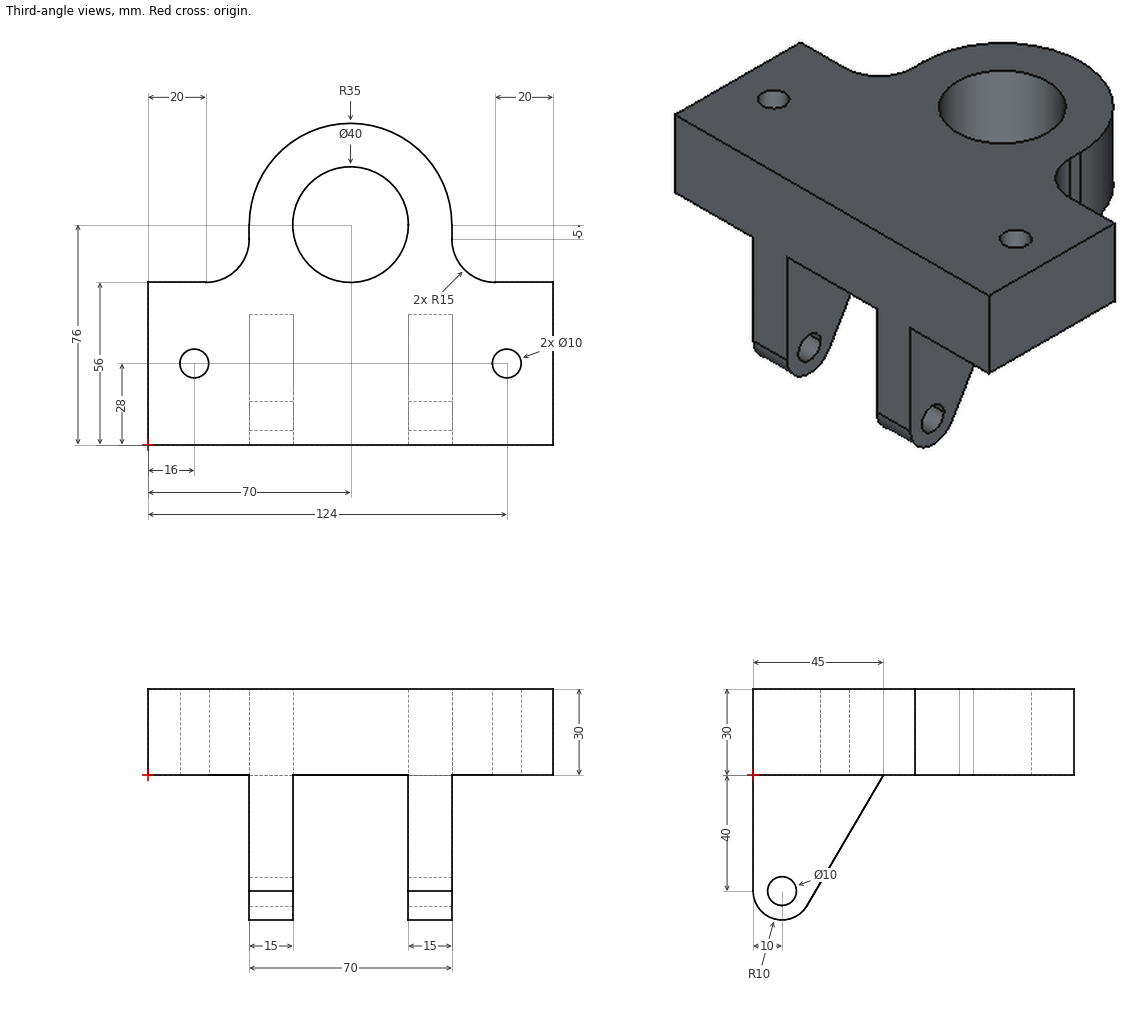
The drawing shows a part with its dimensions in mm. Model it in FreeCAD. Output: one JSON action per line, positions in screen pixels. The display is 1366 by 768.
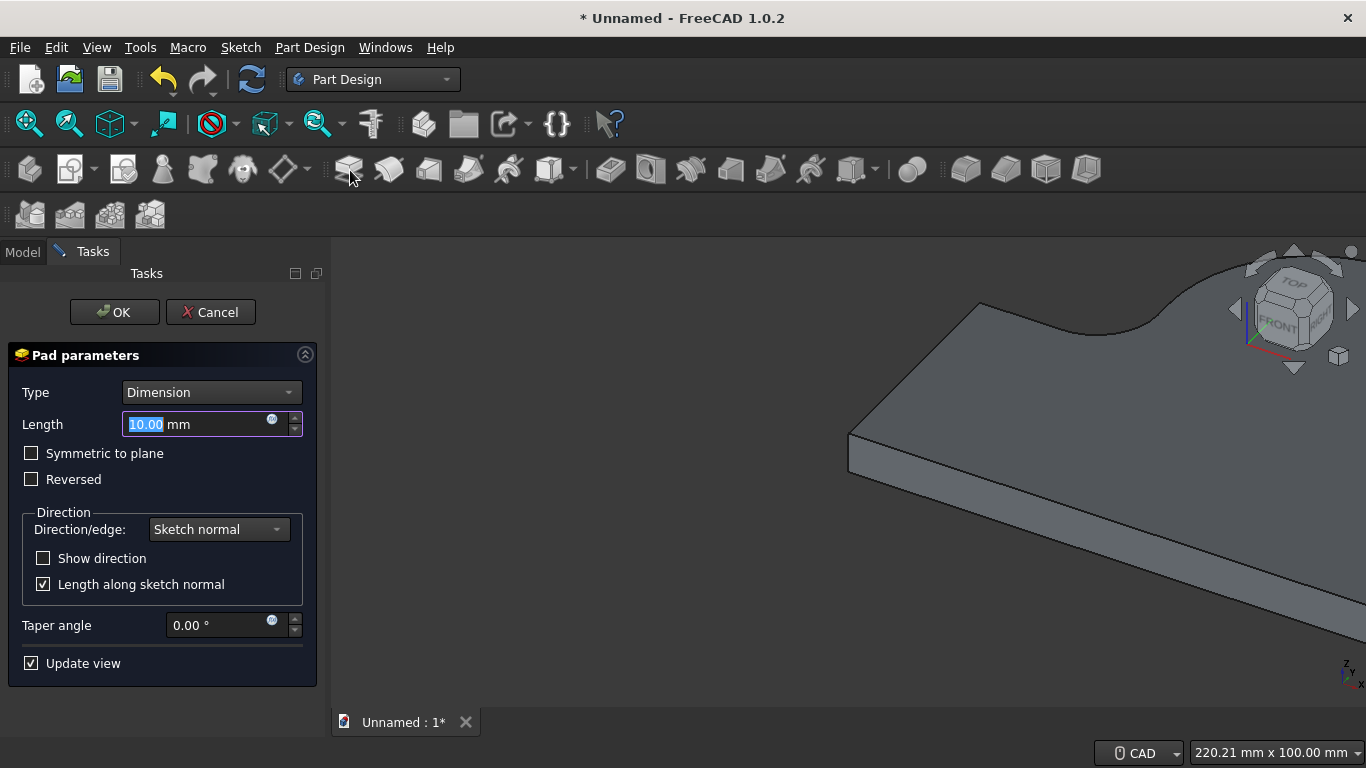
{"action": "type", "text": "30"}
{"action": "key", "text": "Tab"}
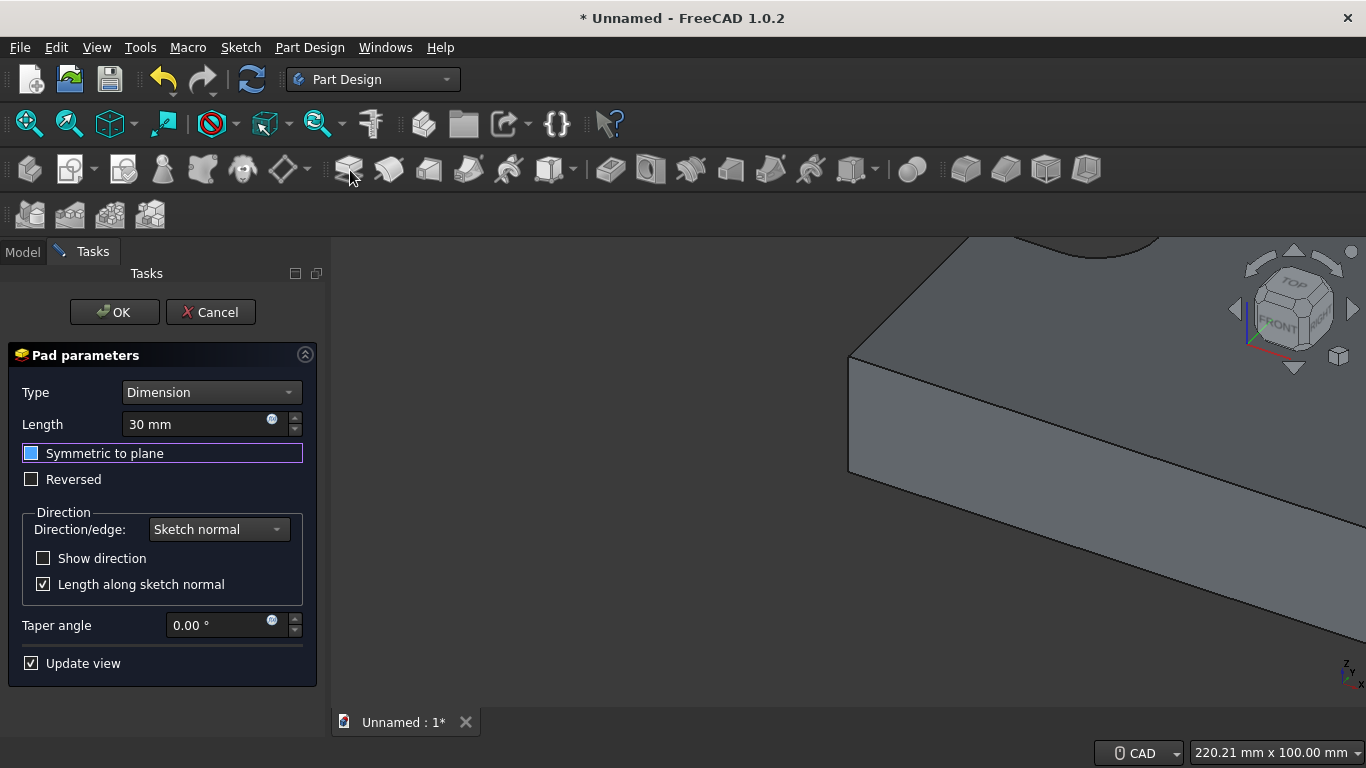
{"action": "left_click", "coordinate": [115, 312]}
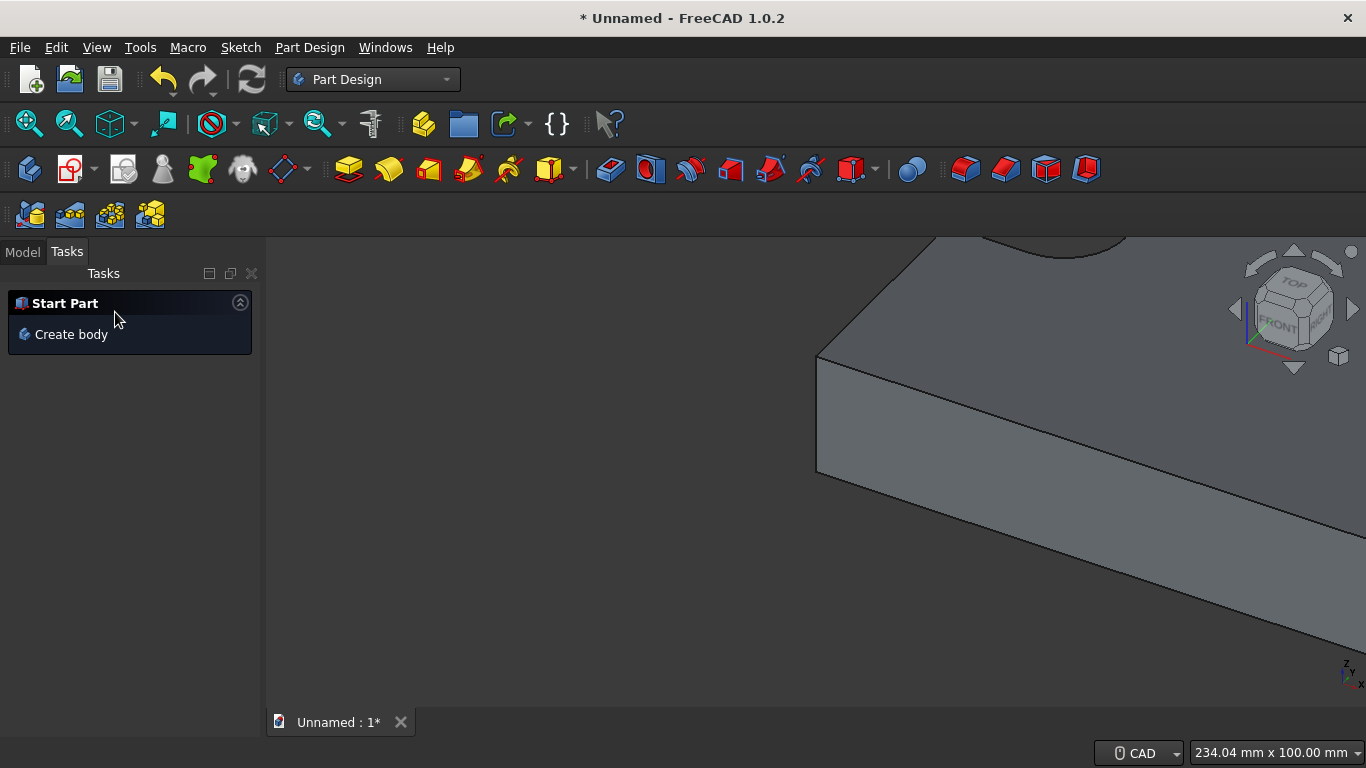
{"action": "left_click", "coordinate": [30, 124]}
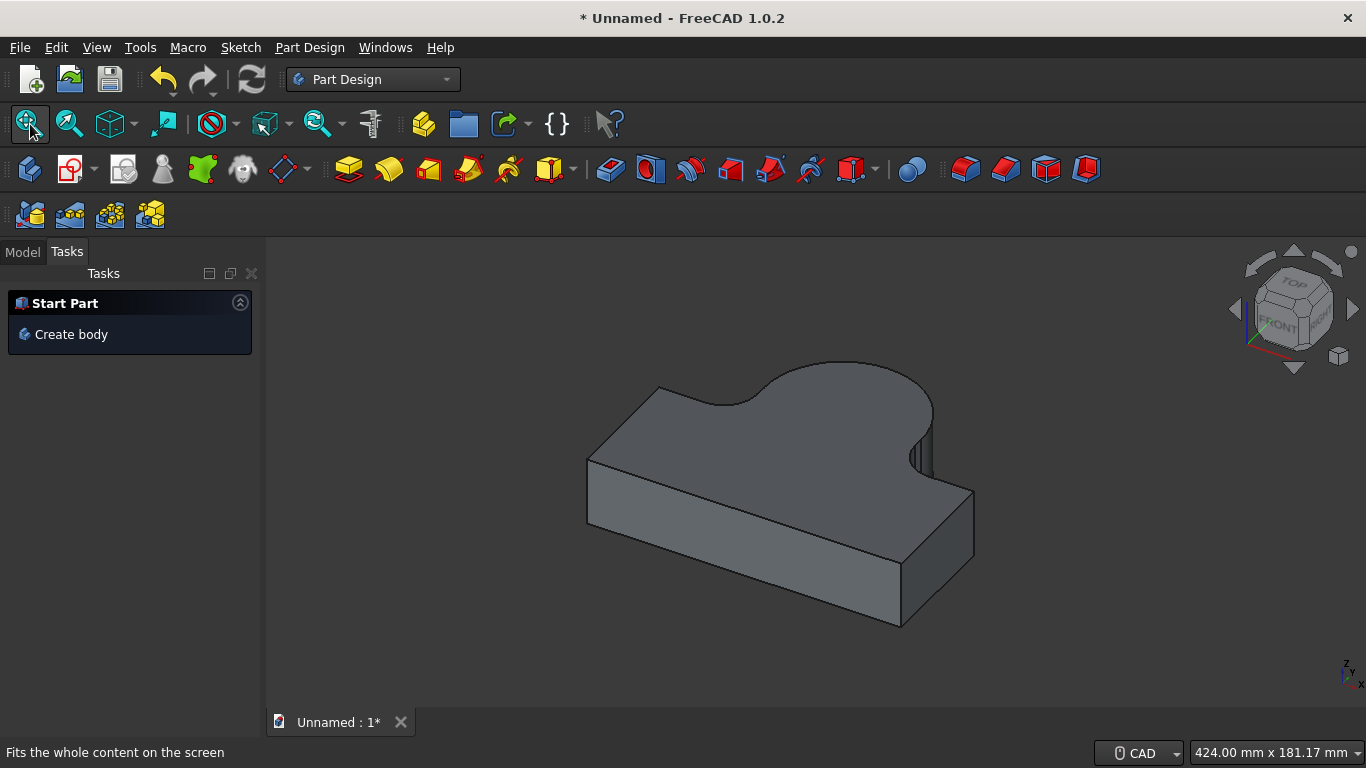
{"action": "left_click", "coordinate": [795, 460]}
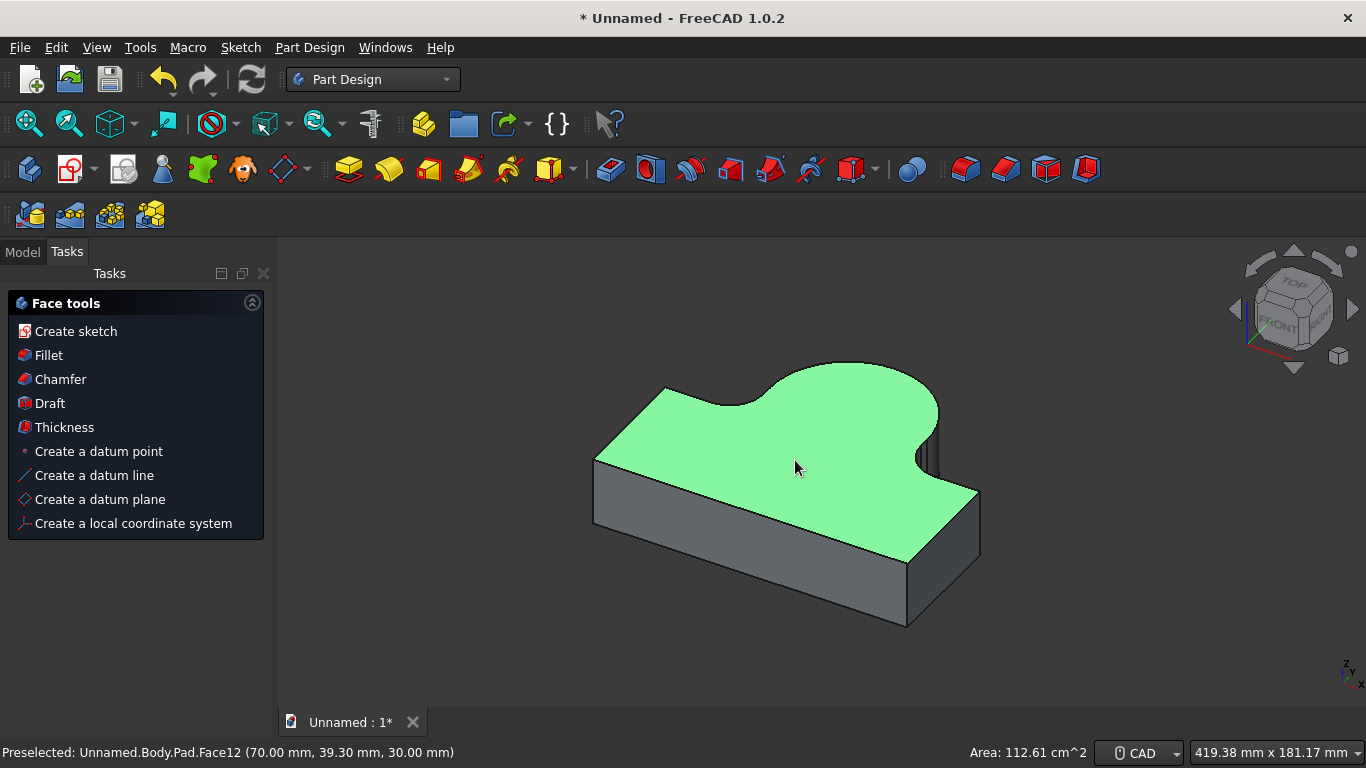
{"action": "left_click", "coordinate": [70, 170]}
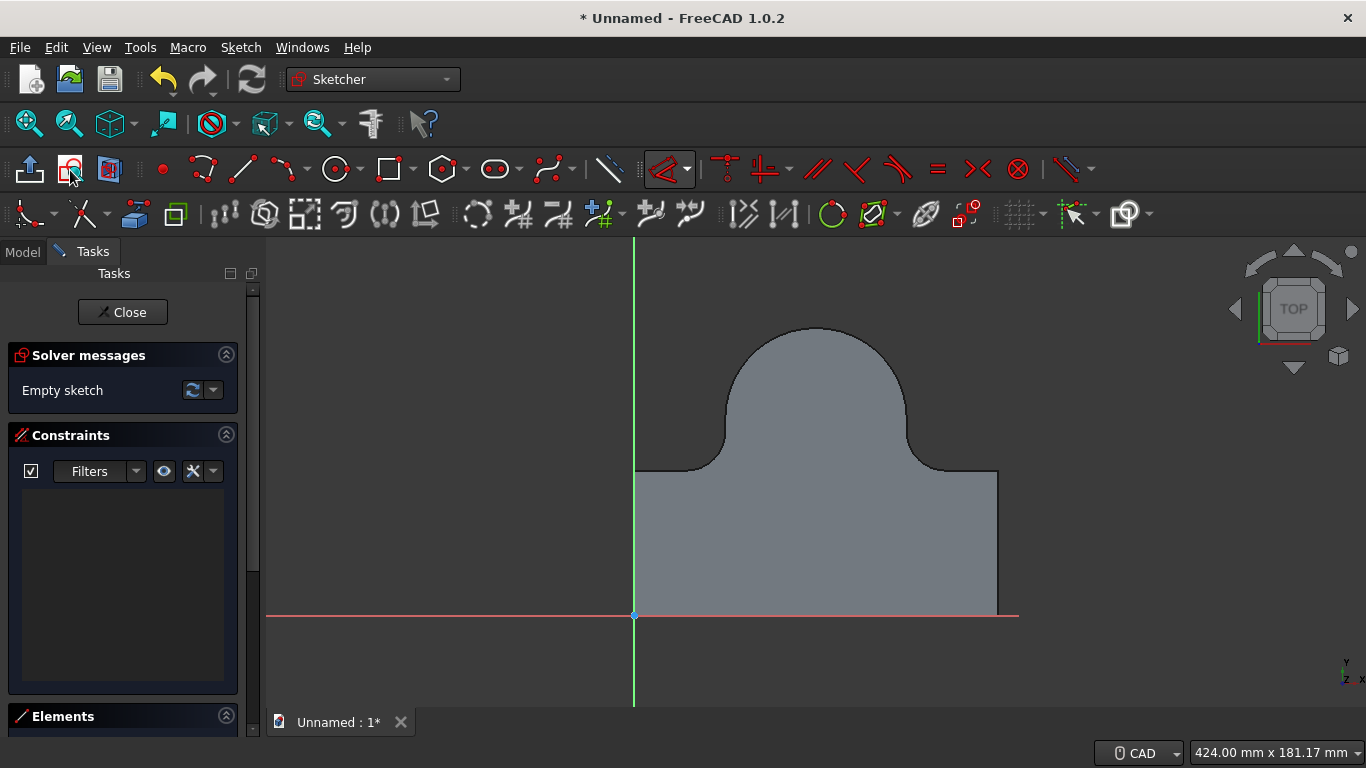
{"action": "left_click", "coordinate": [336, 170]}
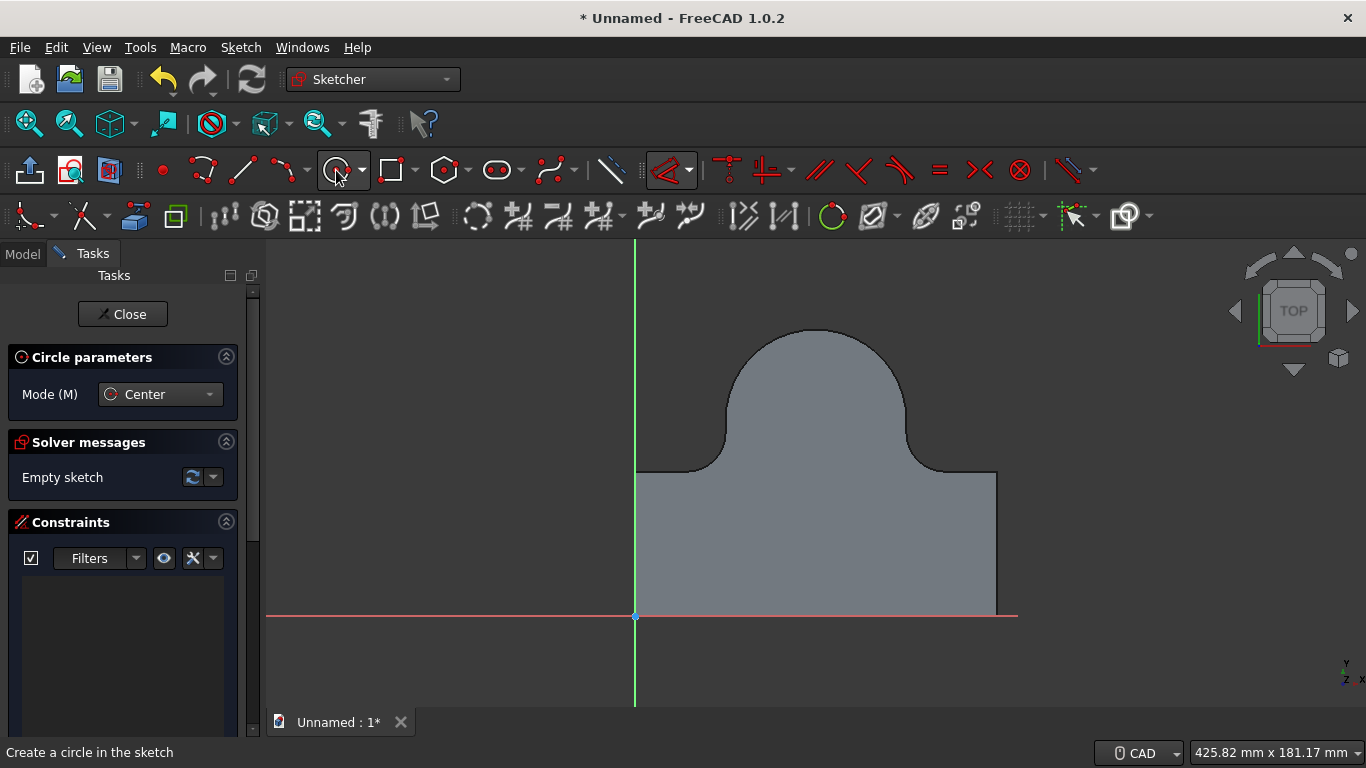
{"action": "left_click", "coordinate": [816, 420]}
{"action": "mouse_move", "coordinate": [853, 384]}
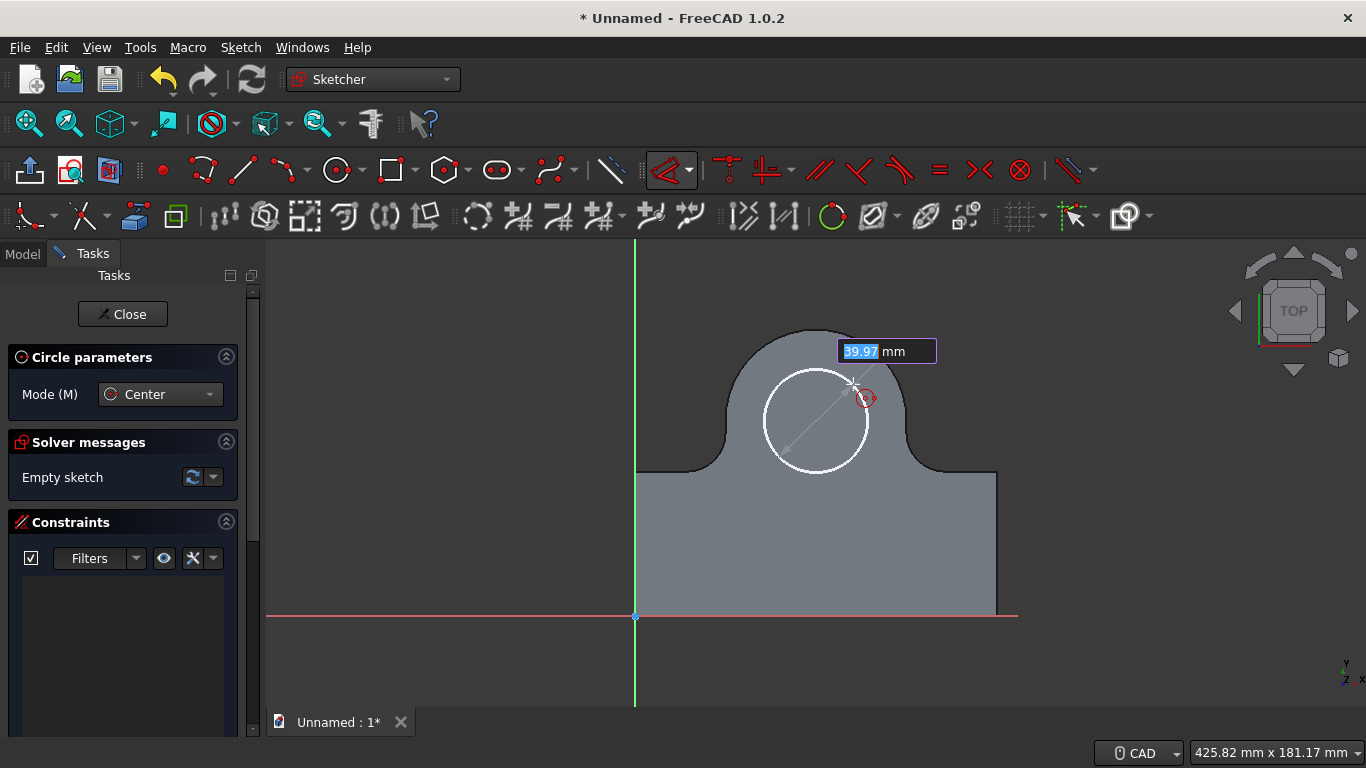
{"action": "type", "text": "40"}
{"action": "key", "text": "Return"}
{"action": "key", "text": "Escape"}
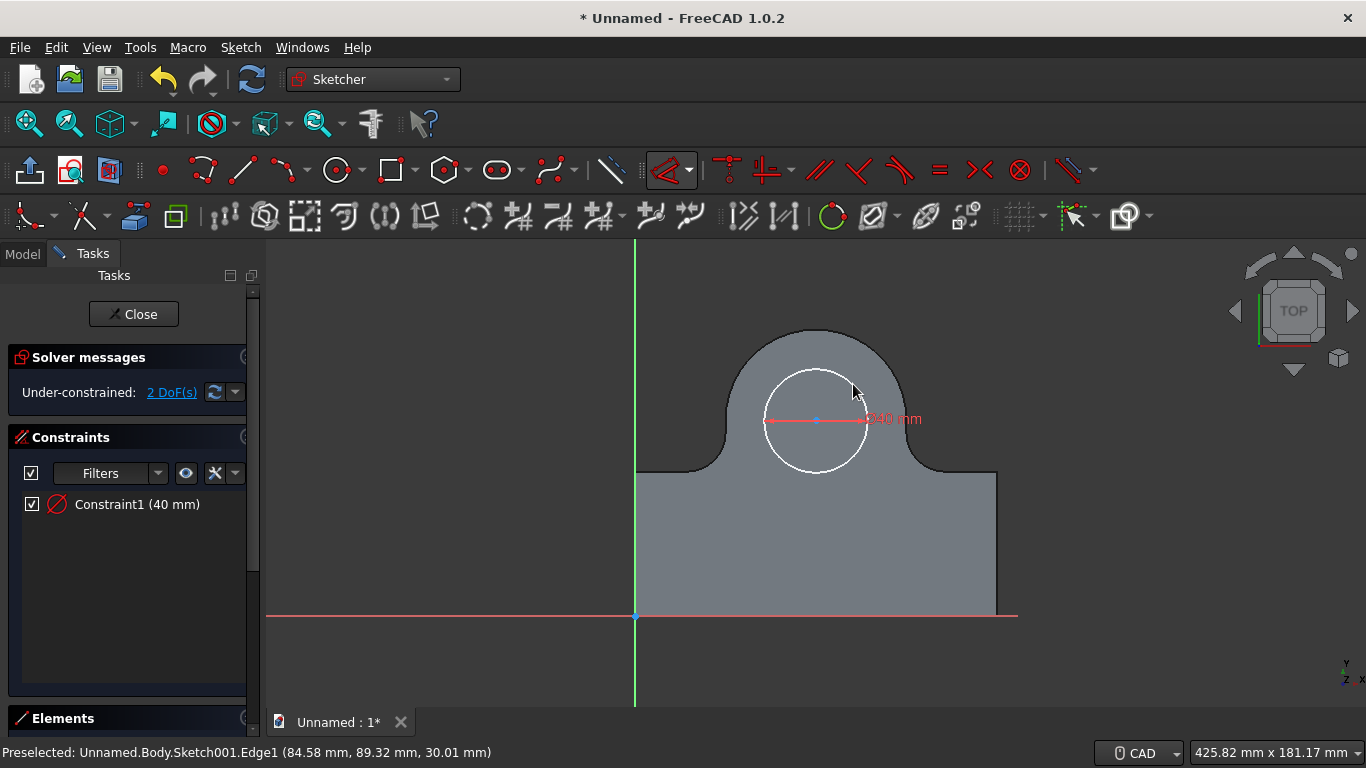
{"action": "left_click", "coordinate": [816, 421]}